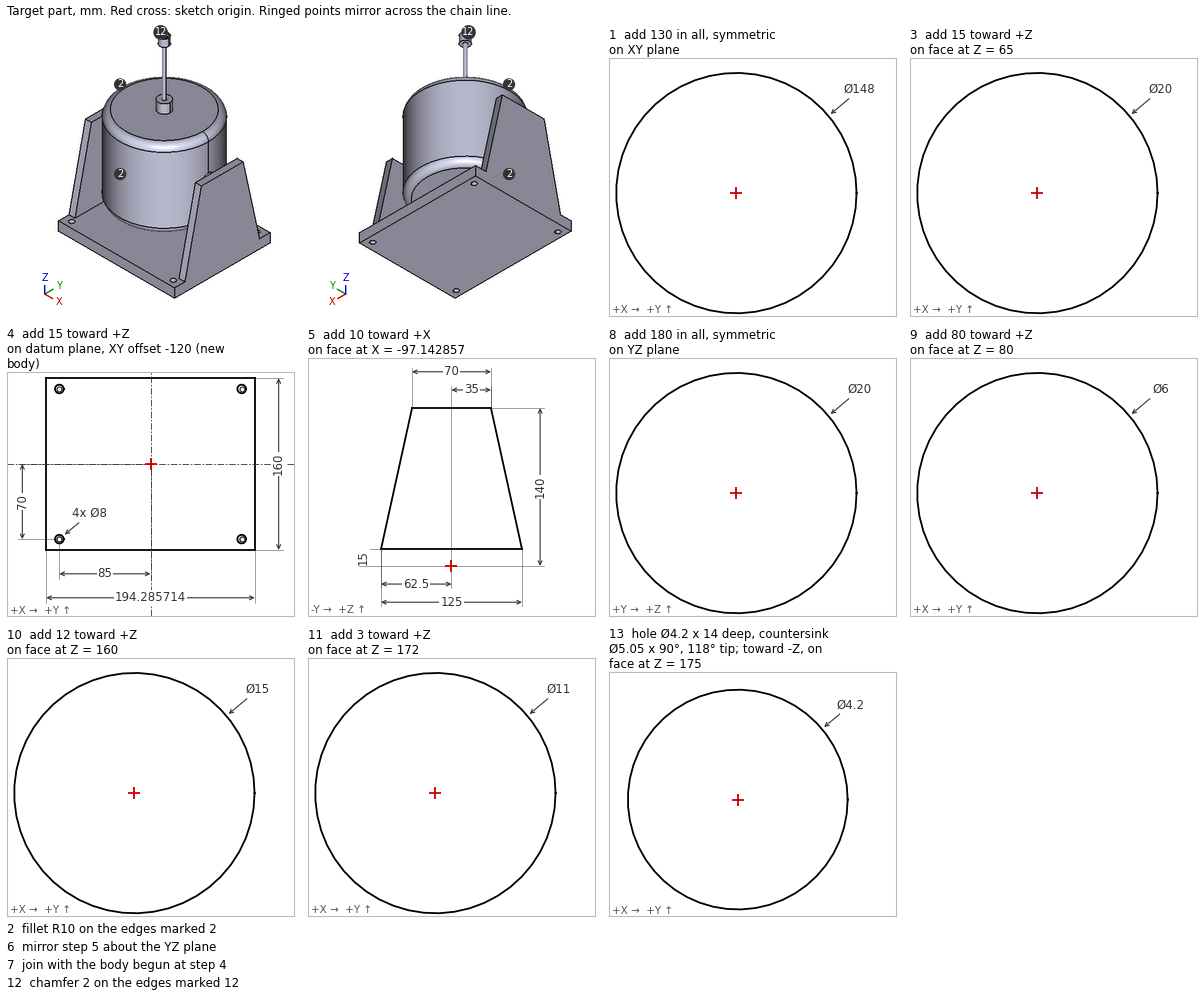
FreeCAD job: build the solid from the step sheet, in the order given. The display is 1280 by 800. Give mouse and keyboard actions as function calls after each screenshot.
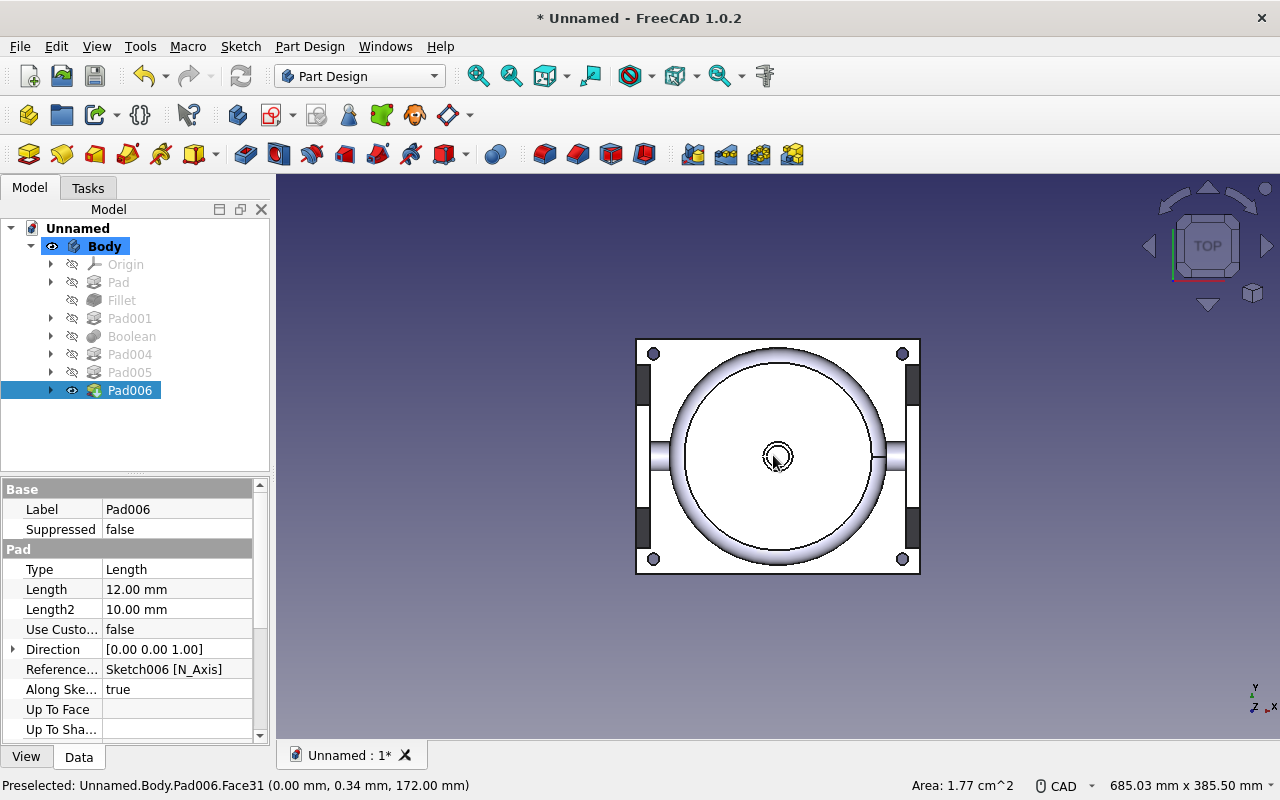
click(270, 116)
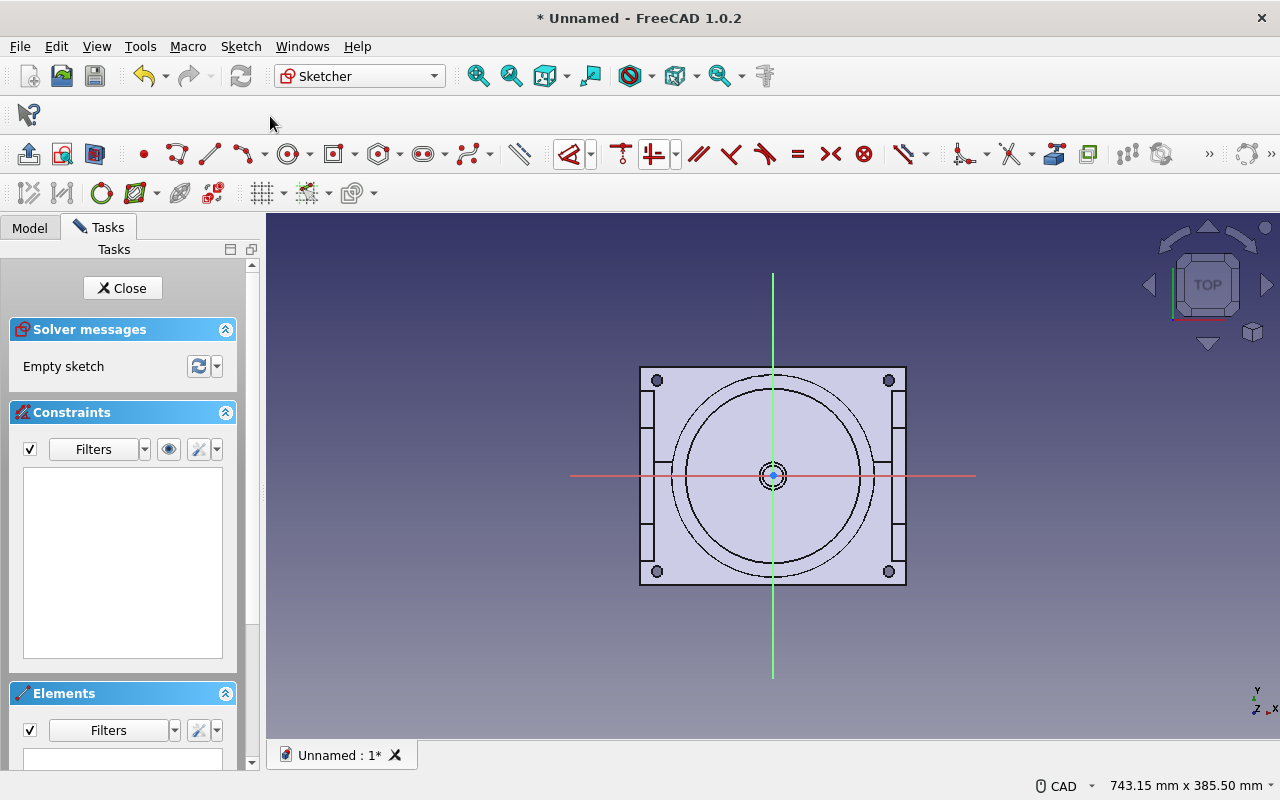
scroll(777, 476, up, 15)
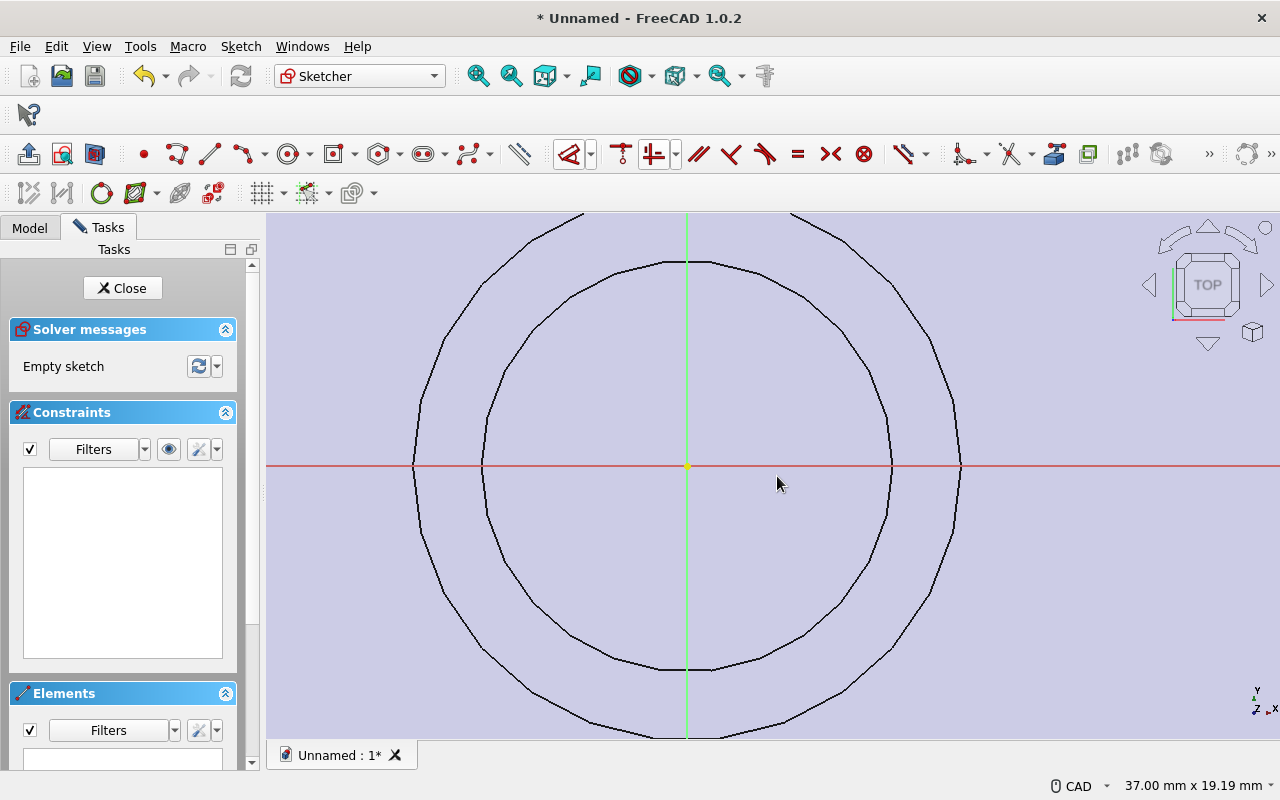
key(g)
key(c)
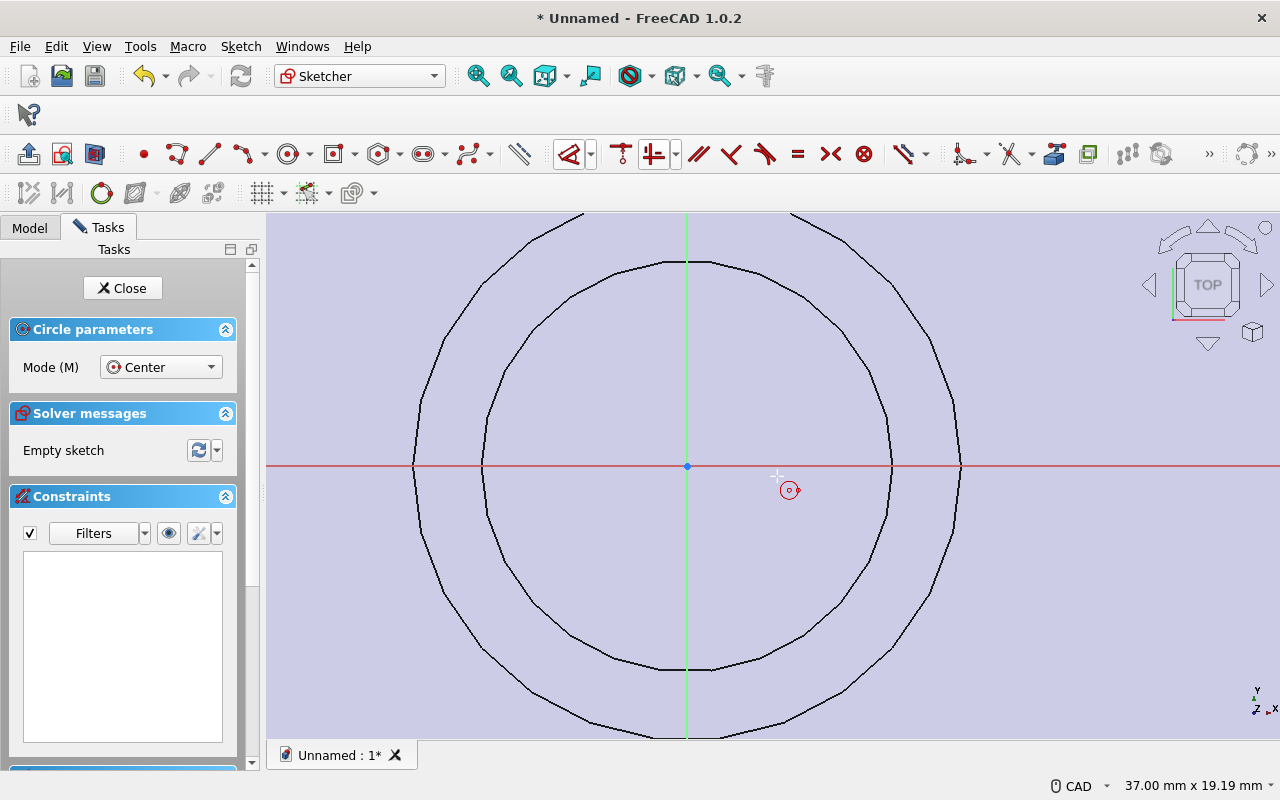
click(687, 466)
click(794, 360)
key(Escape)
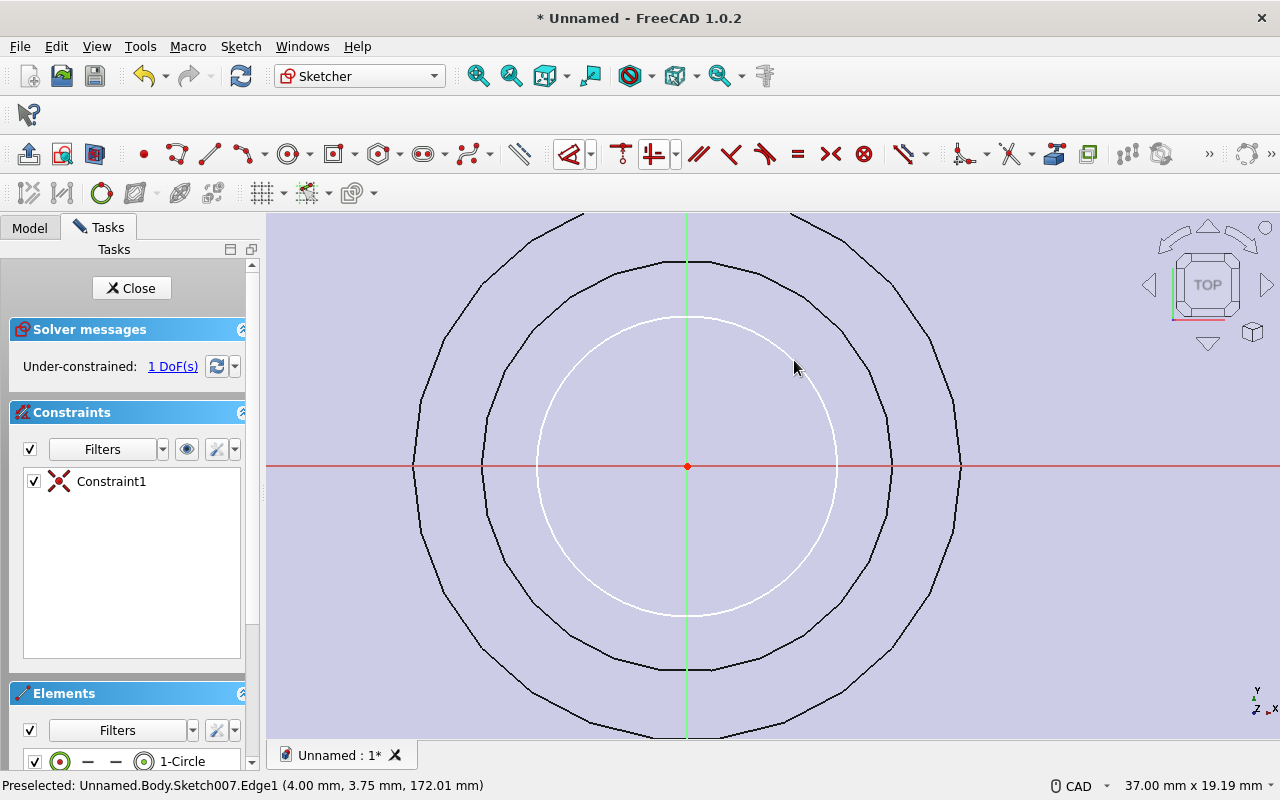
click(793, 360)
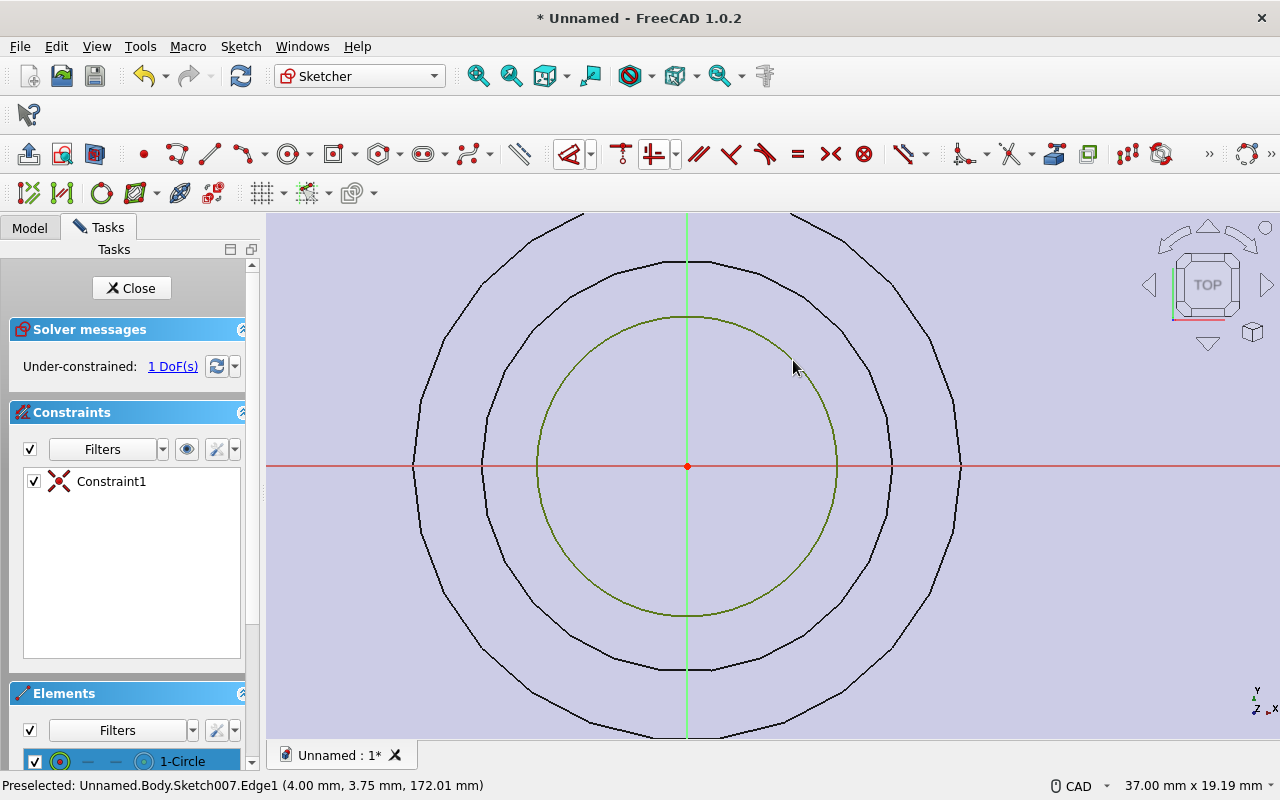
key(k)
key(o)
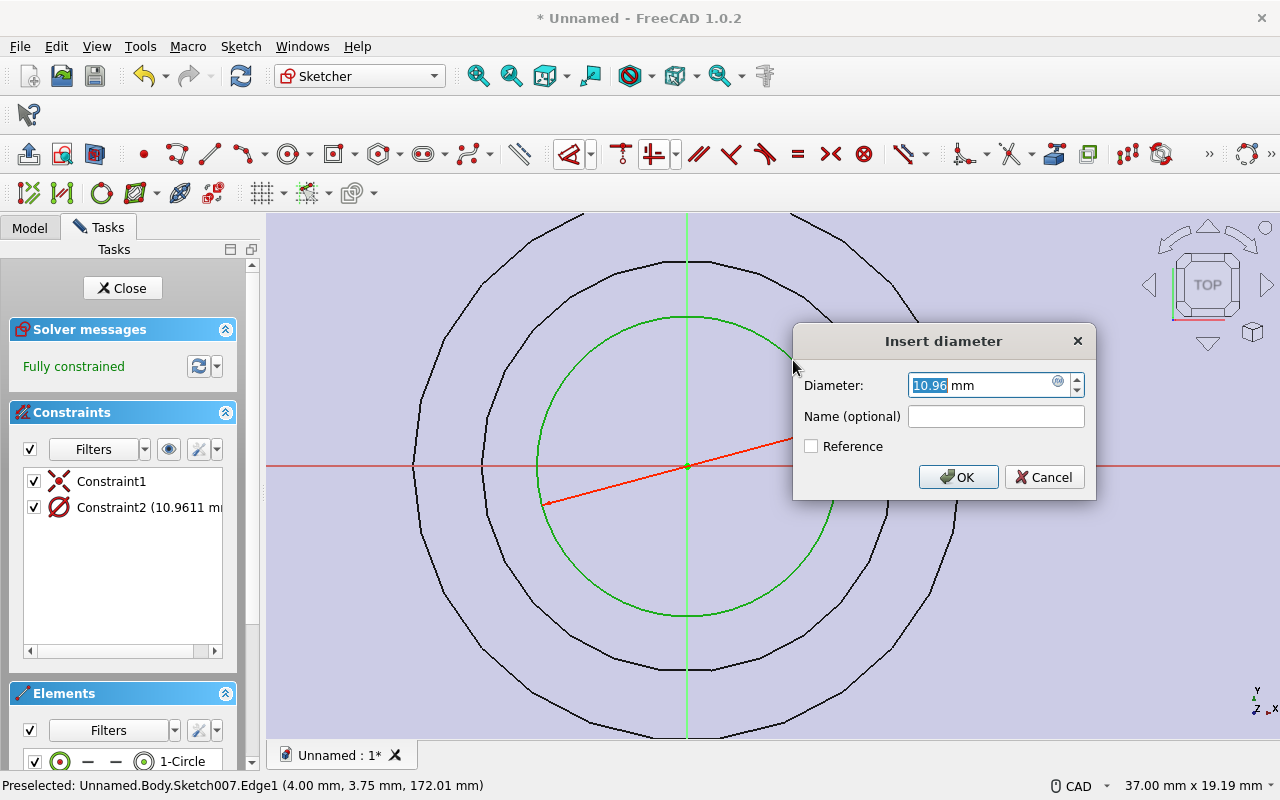
text(11)
key(Return)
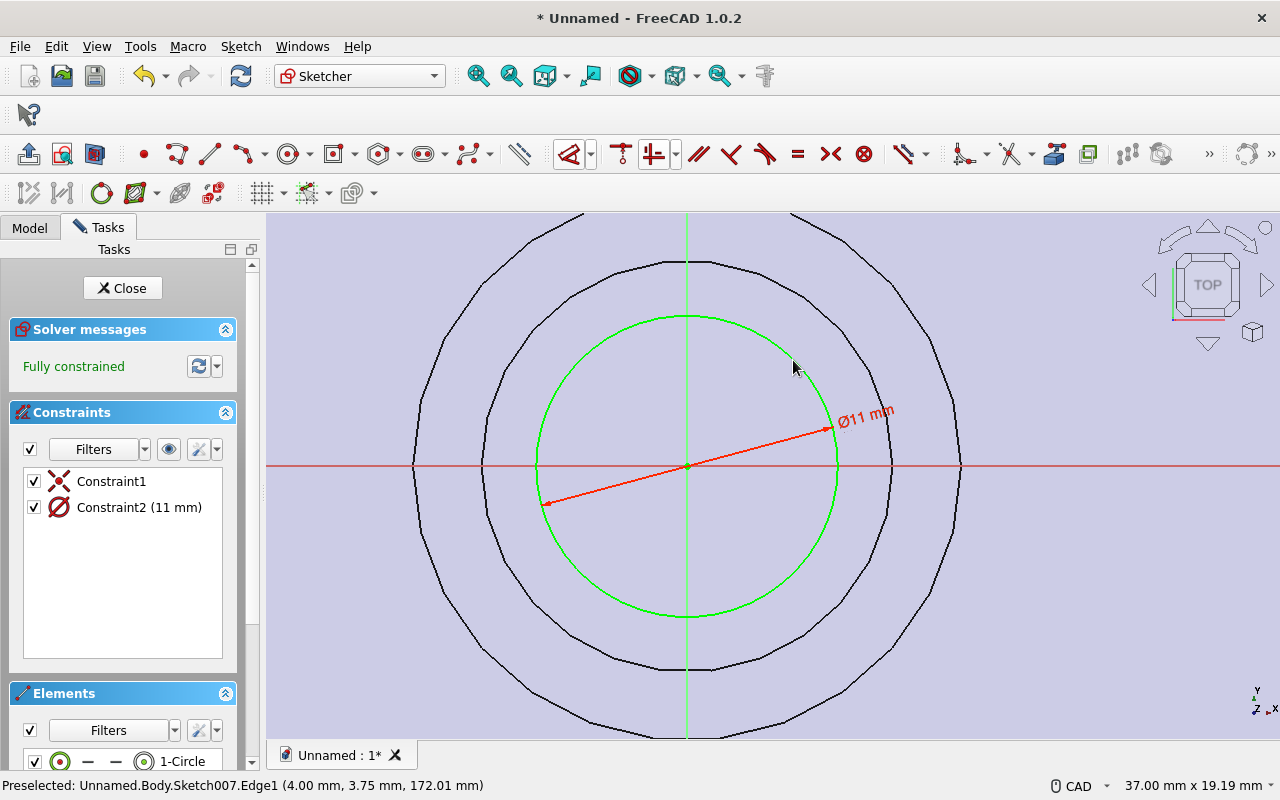
click(123, 288)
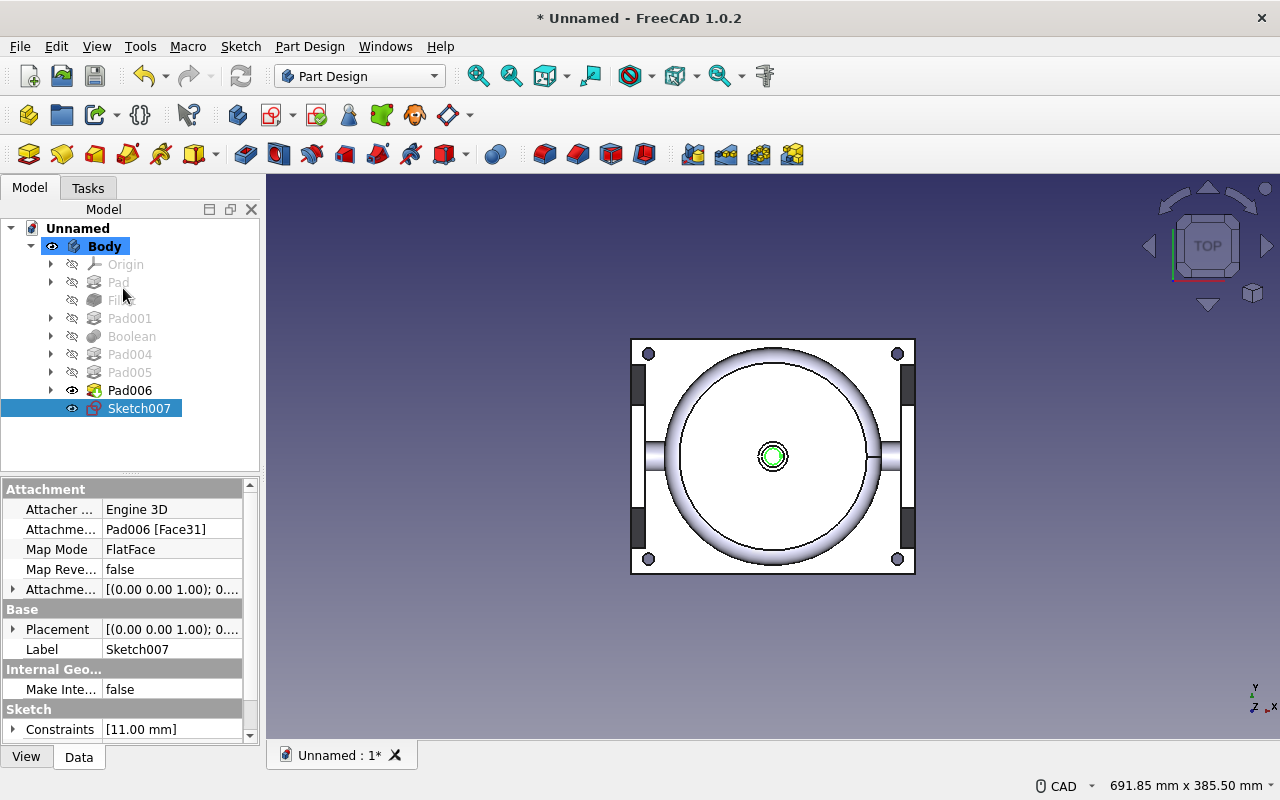
click(29, 154)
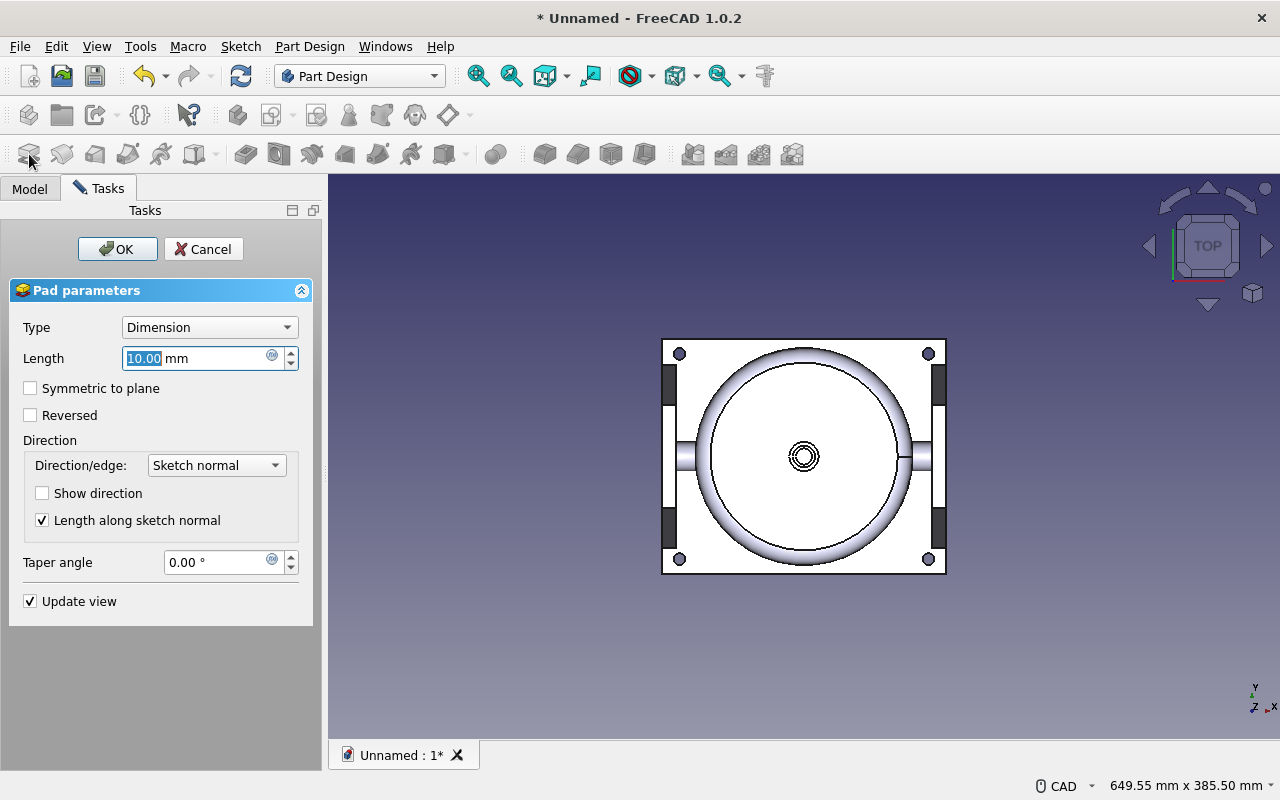
text(3)
key(Tab)